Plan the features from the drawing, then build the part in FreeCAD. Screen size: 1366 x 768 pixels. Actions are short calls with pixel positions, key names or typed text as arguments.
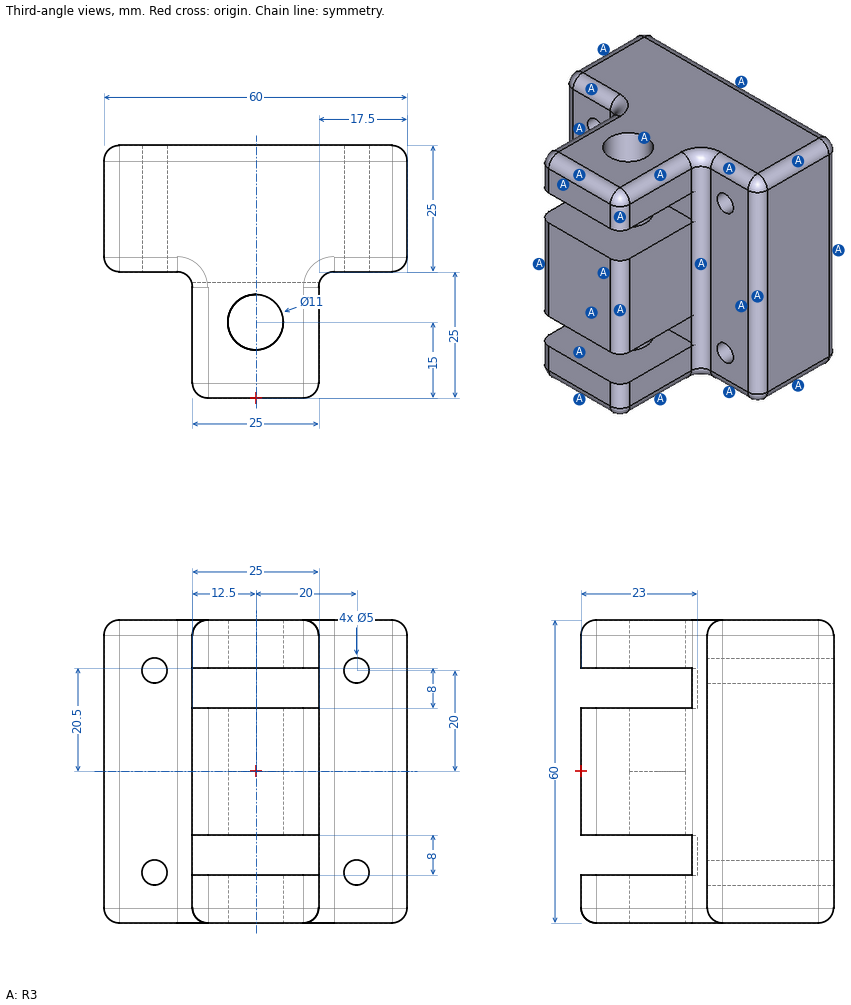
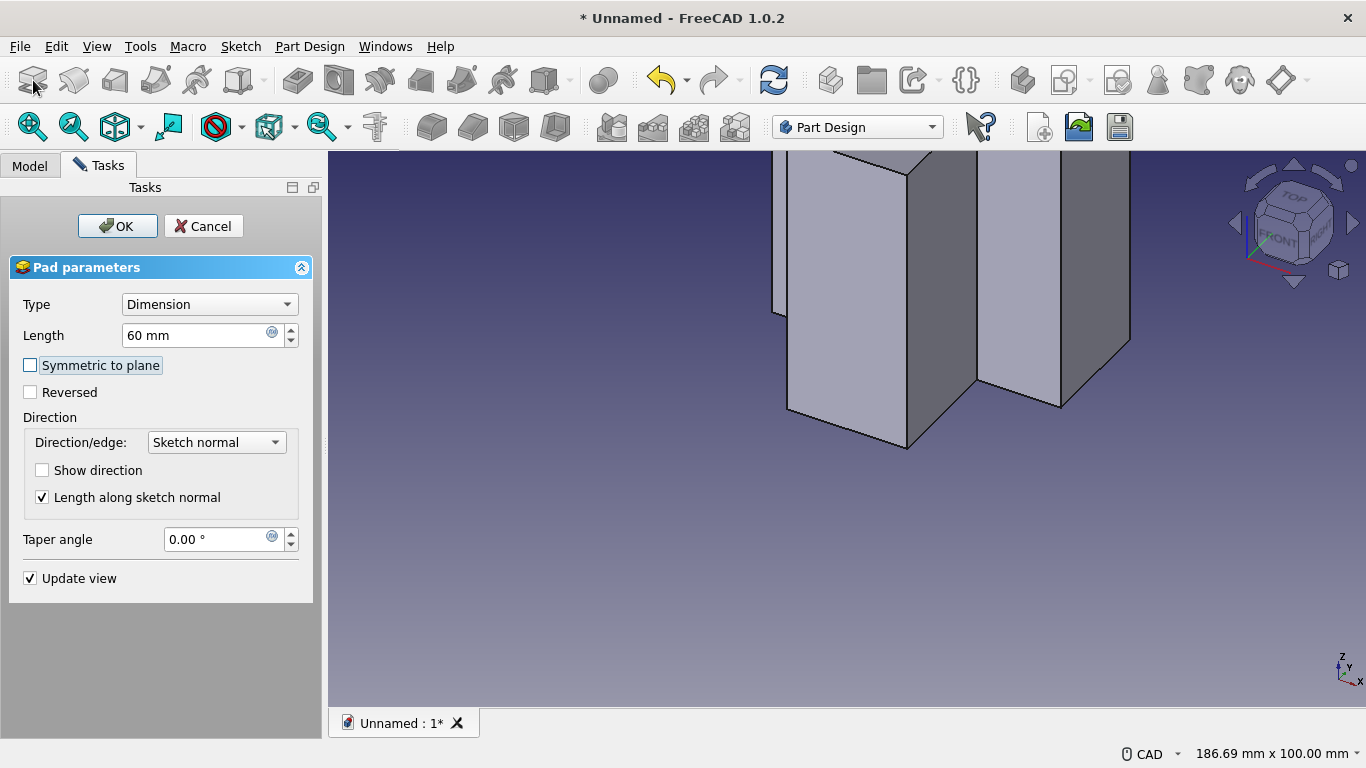
click(31, 365)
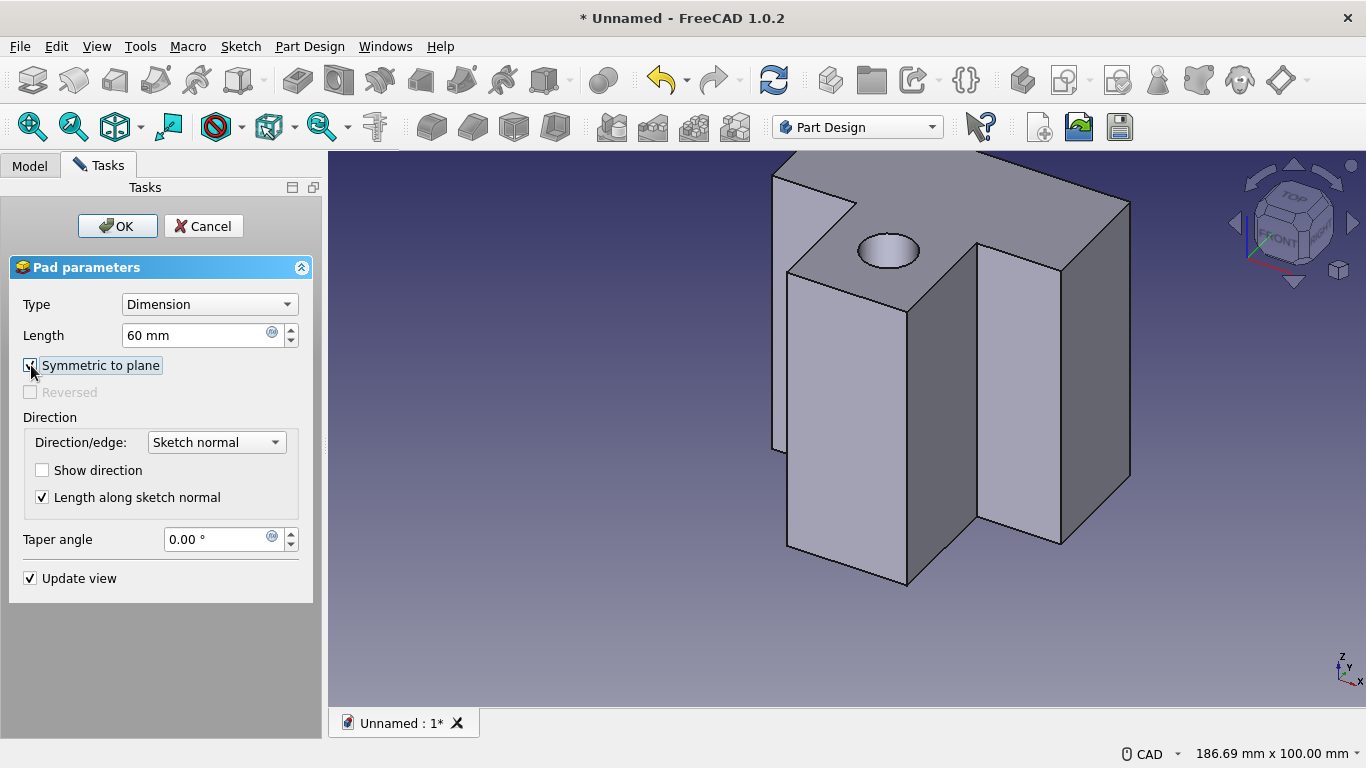
click(118, 226)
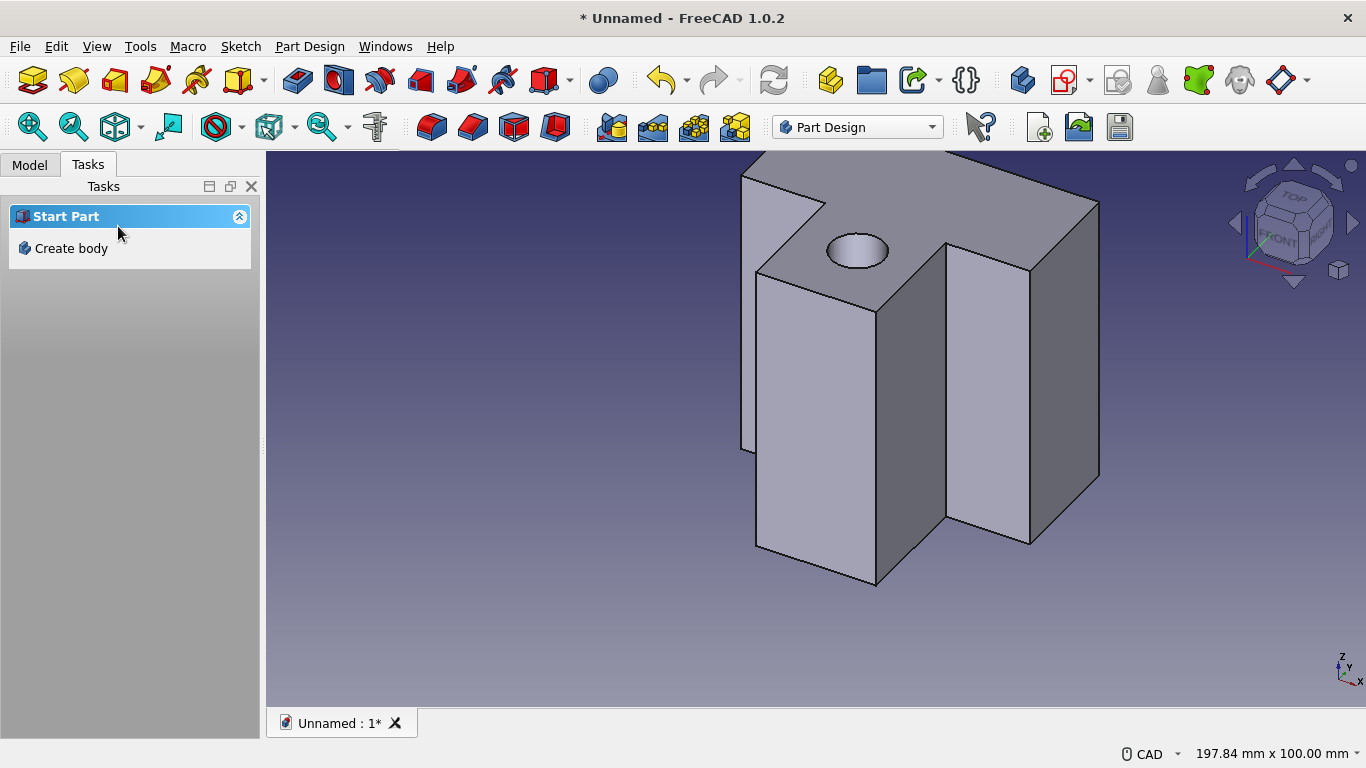
click(33, 128)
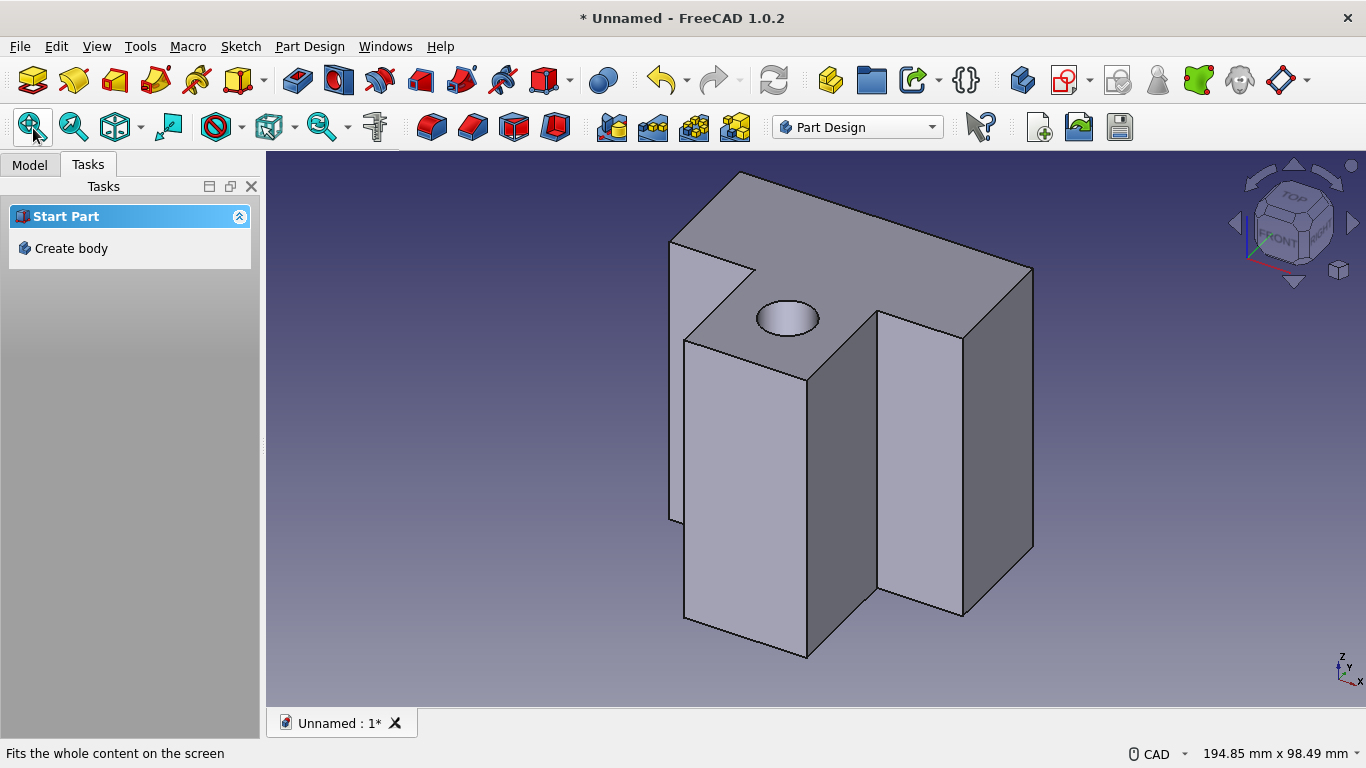
click(745, 419)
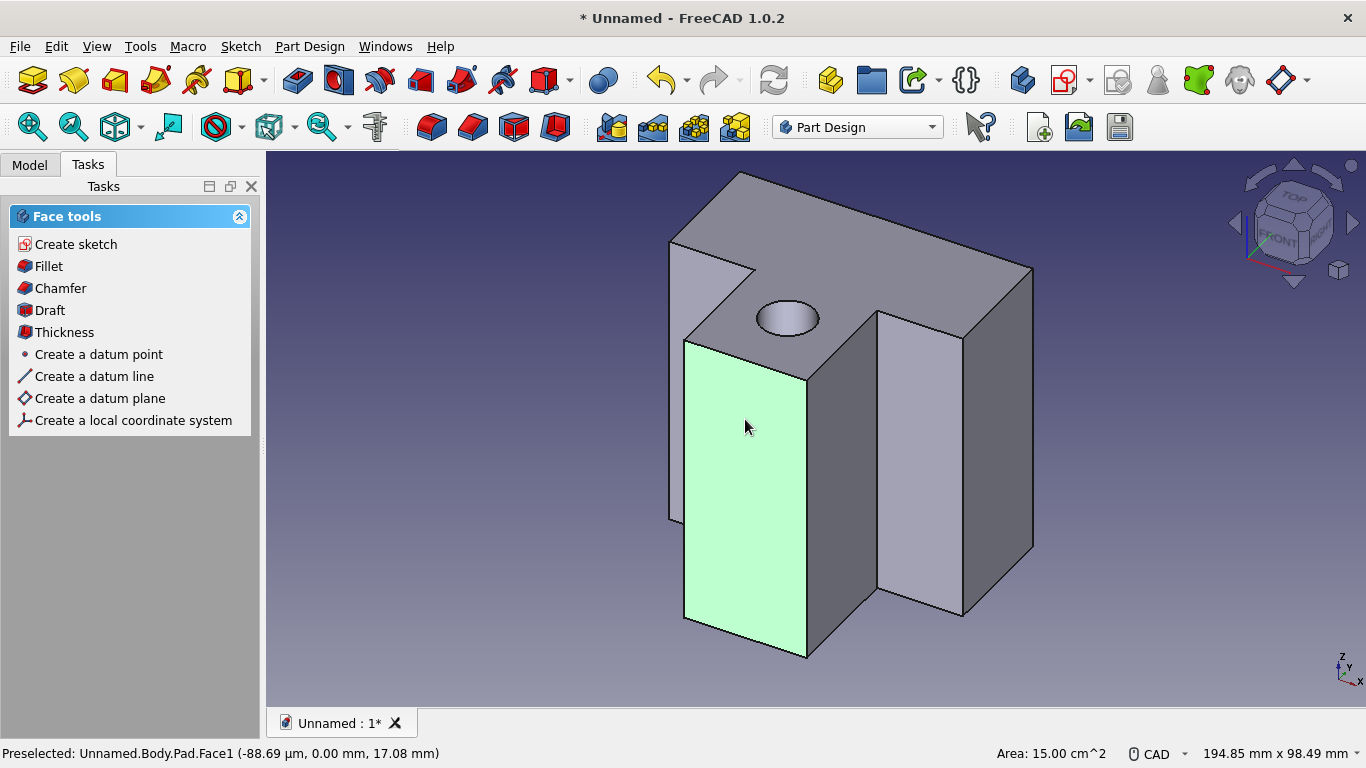
click(847, 404, ctrl)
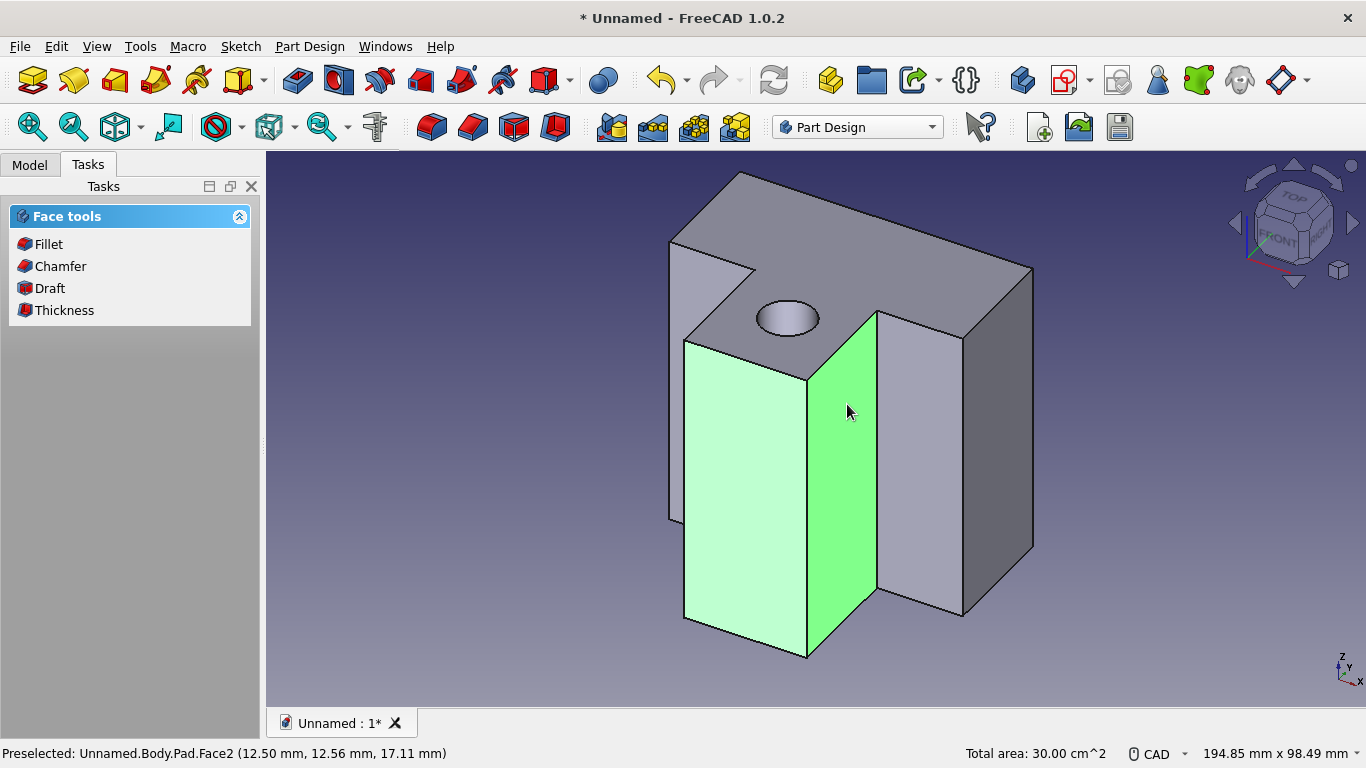
click(998, 362, ctrl)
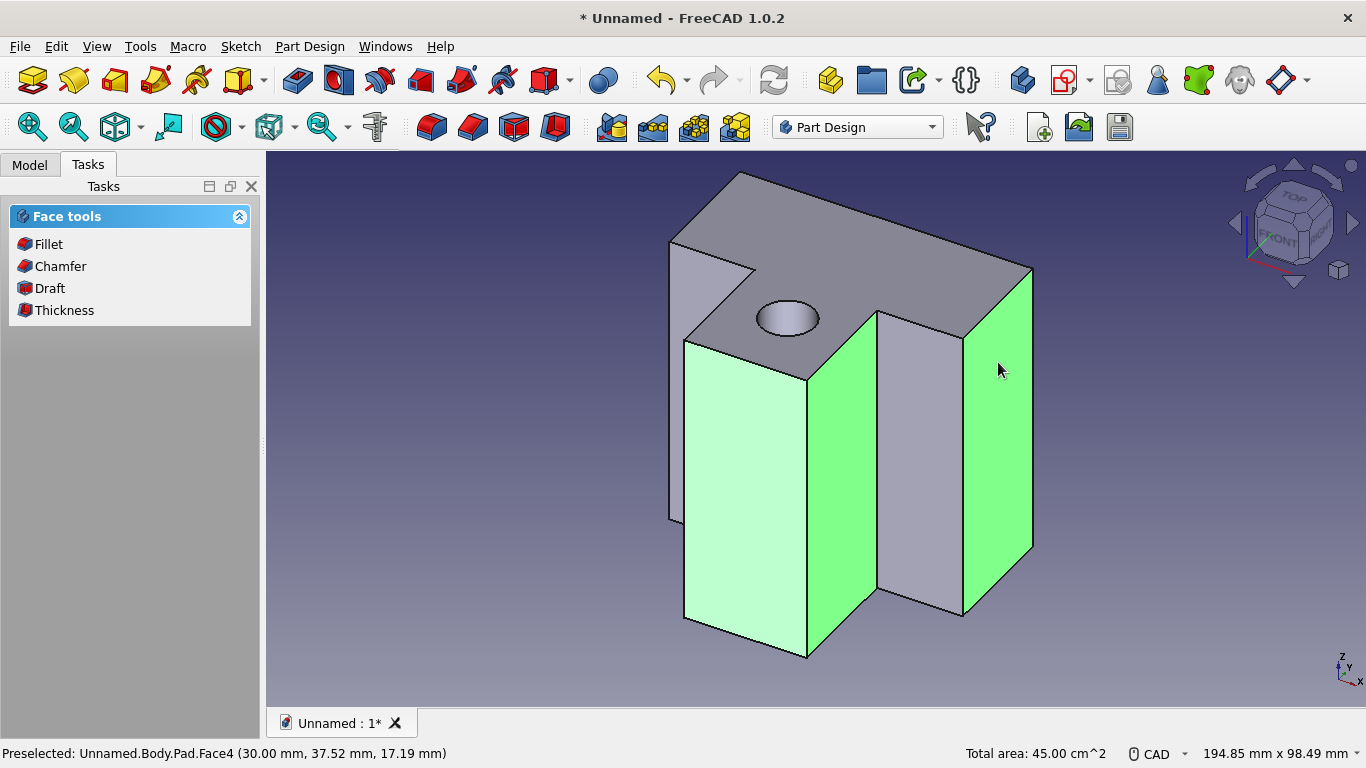
click(712, 255, ctrl)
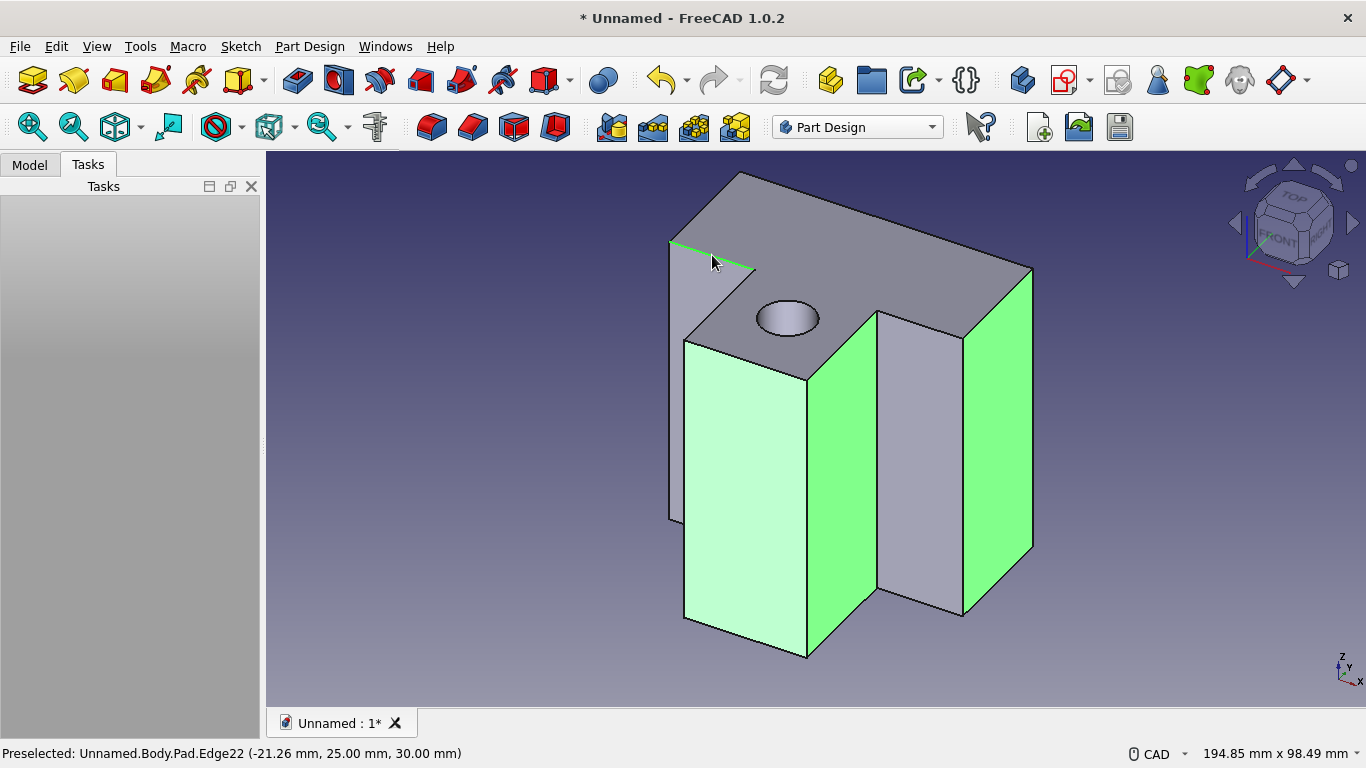
click(920, 324, ctrl)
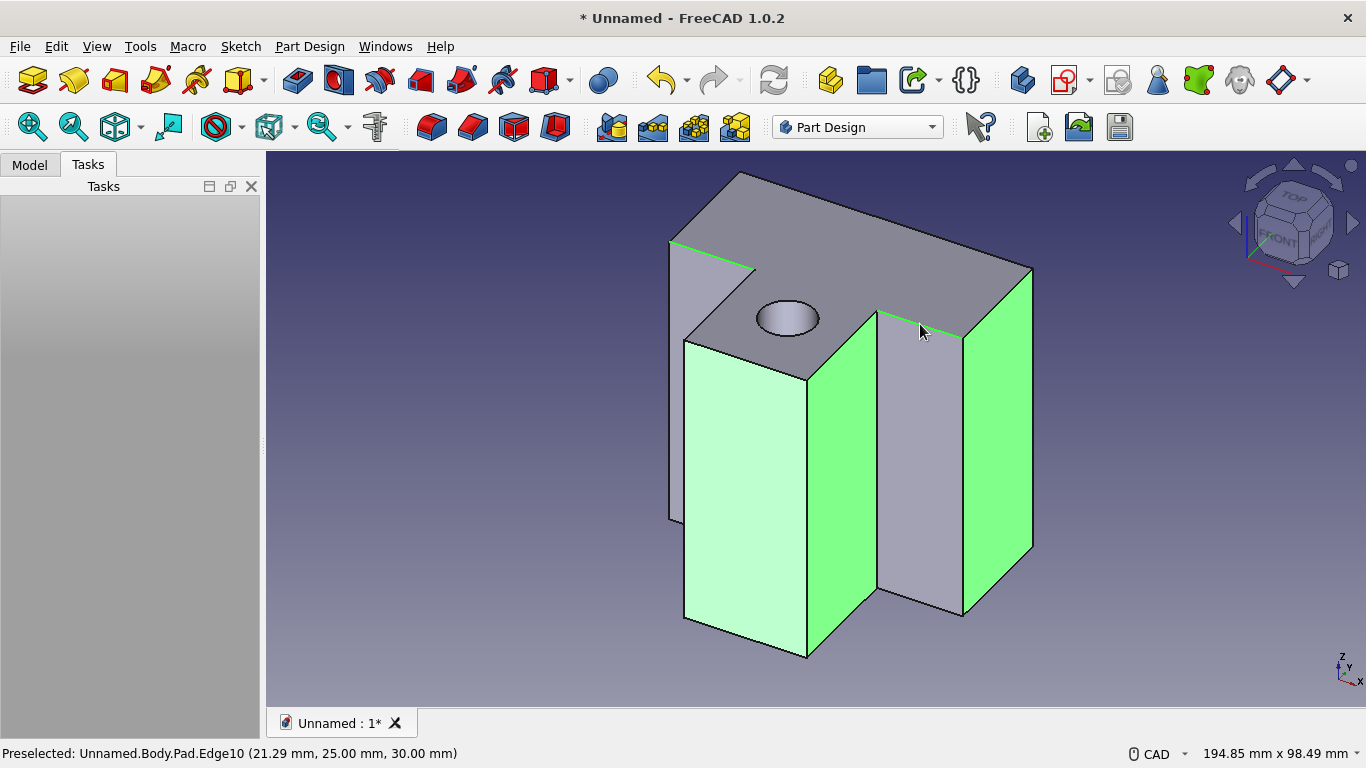
key(0)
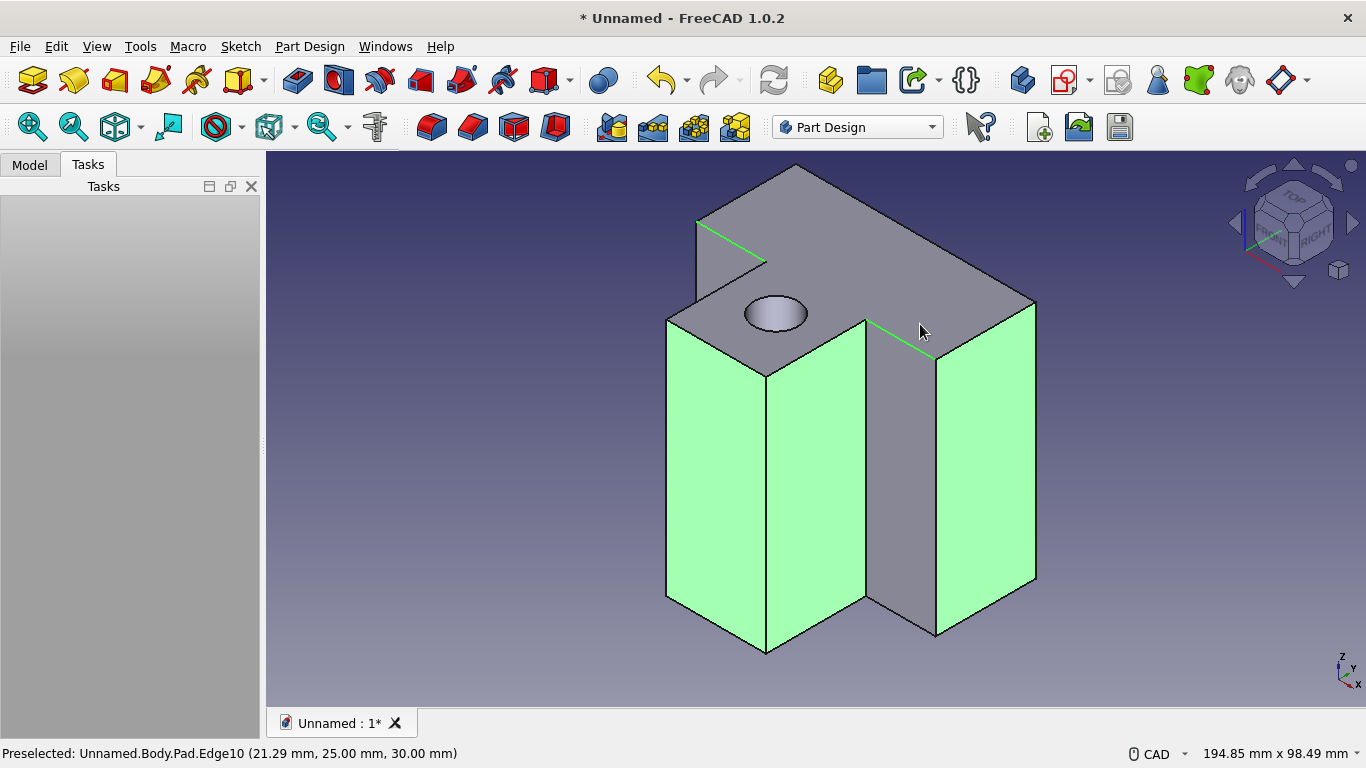
key(2)